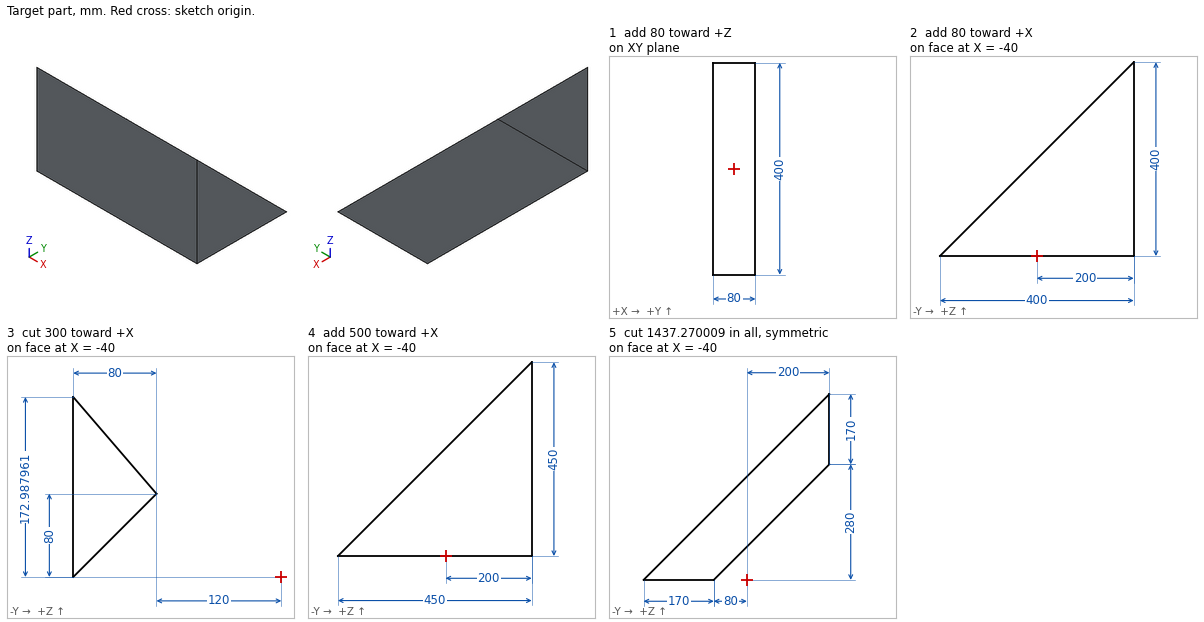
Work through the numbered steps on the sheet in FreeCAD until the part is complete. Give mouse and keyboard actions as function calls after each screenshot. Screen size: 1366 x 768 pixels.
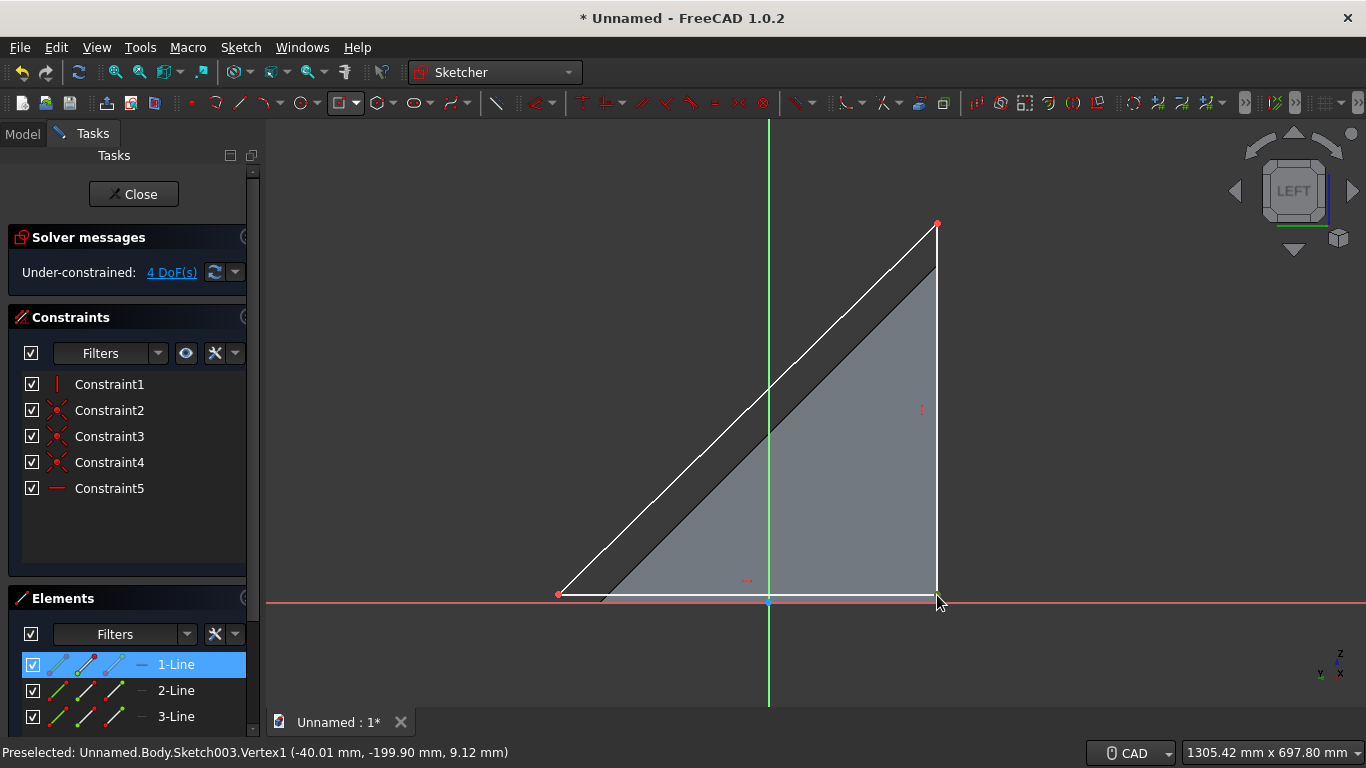
click(359, 603)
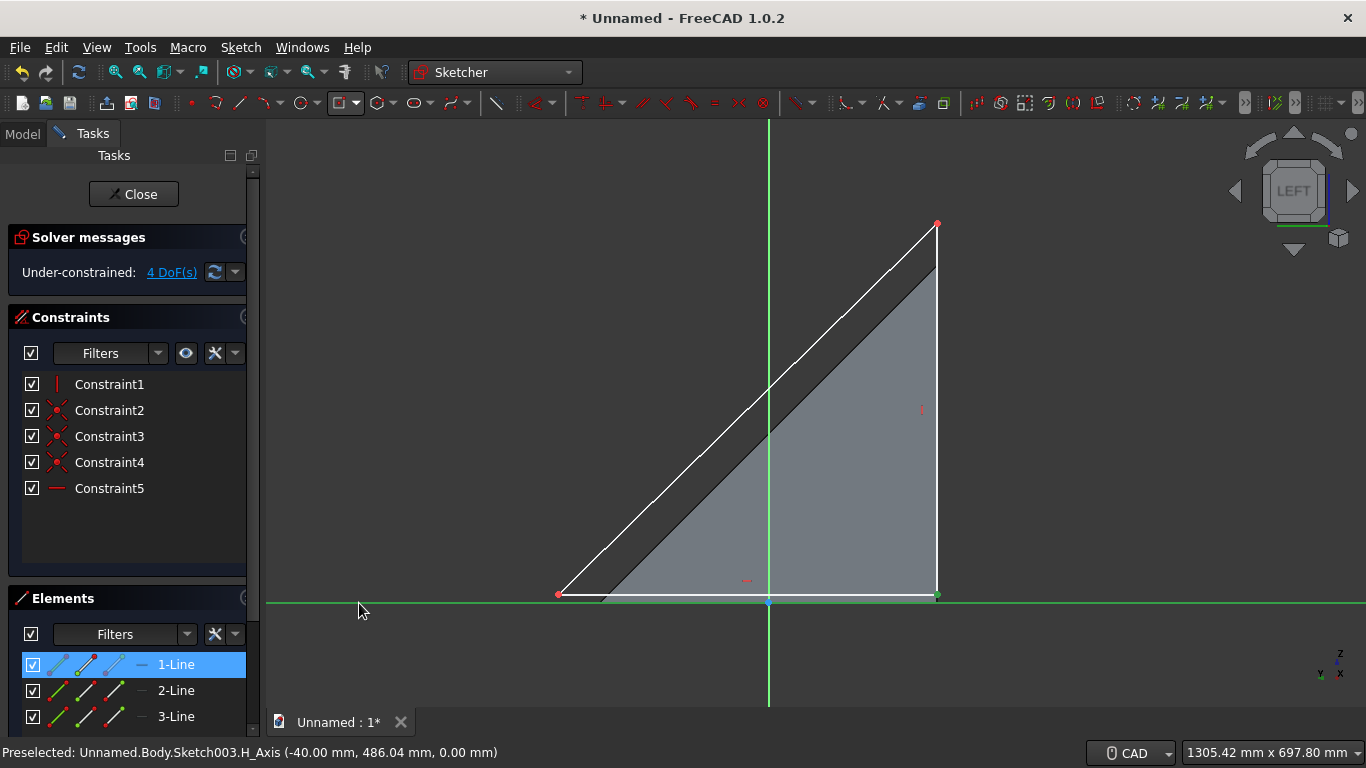
click(582, 104)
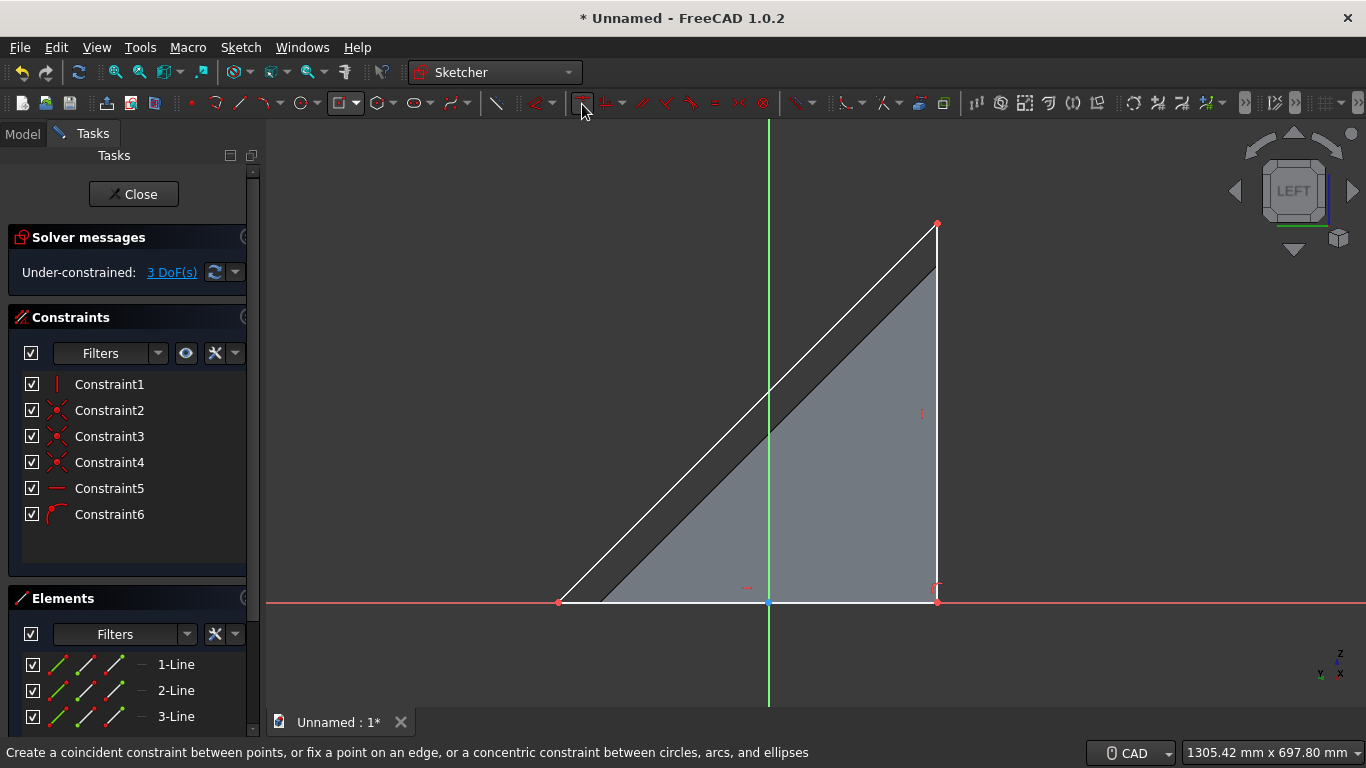
click(536, 104)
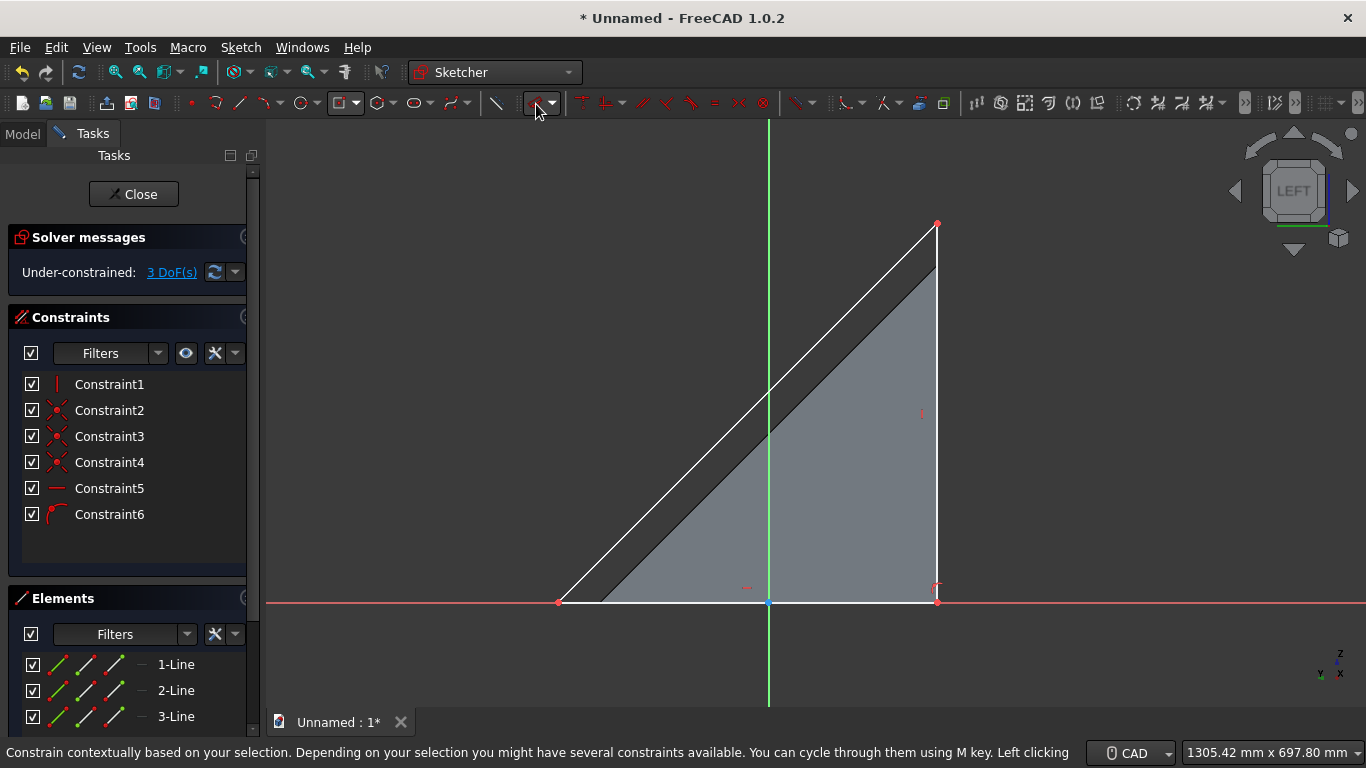
click(937, 489)
click(971, 413)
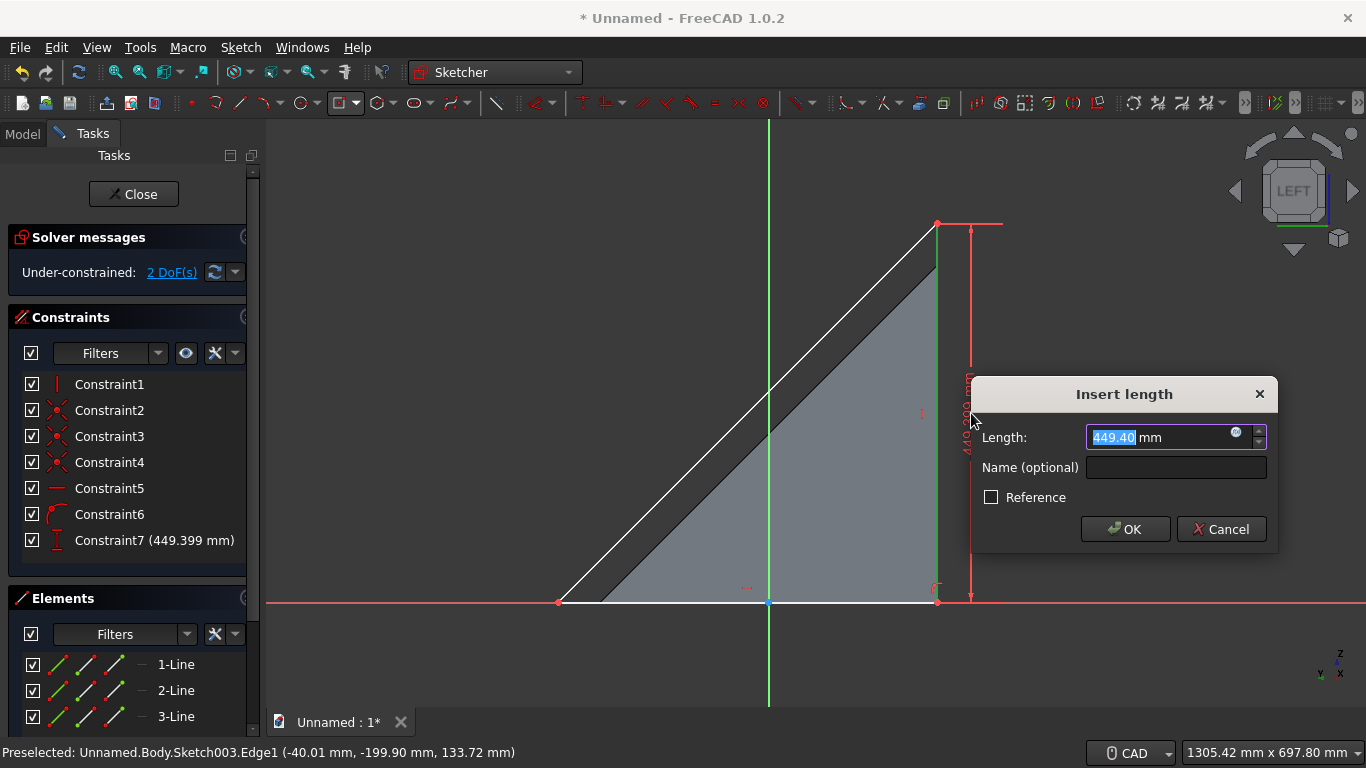
text(450)
key(Return)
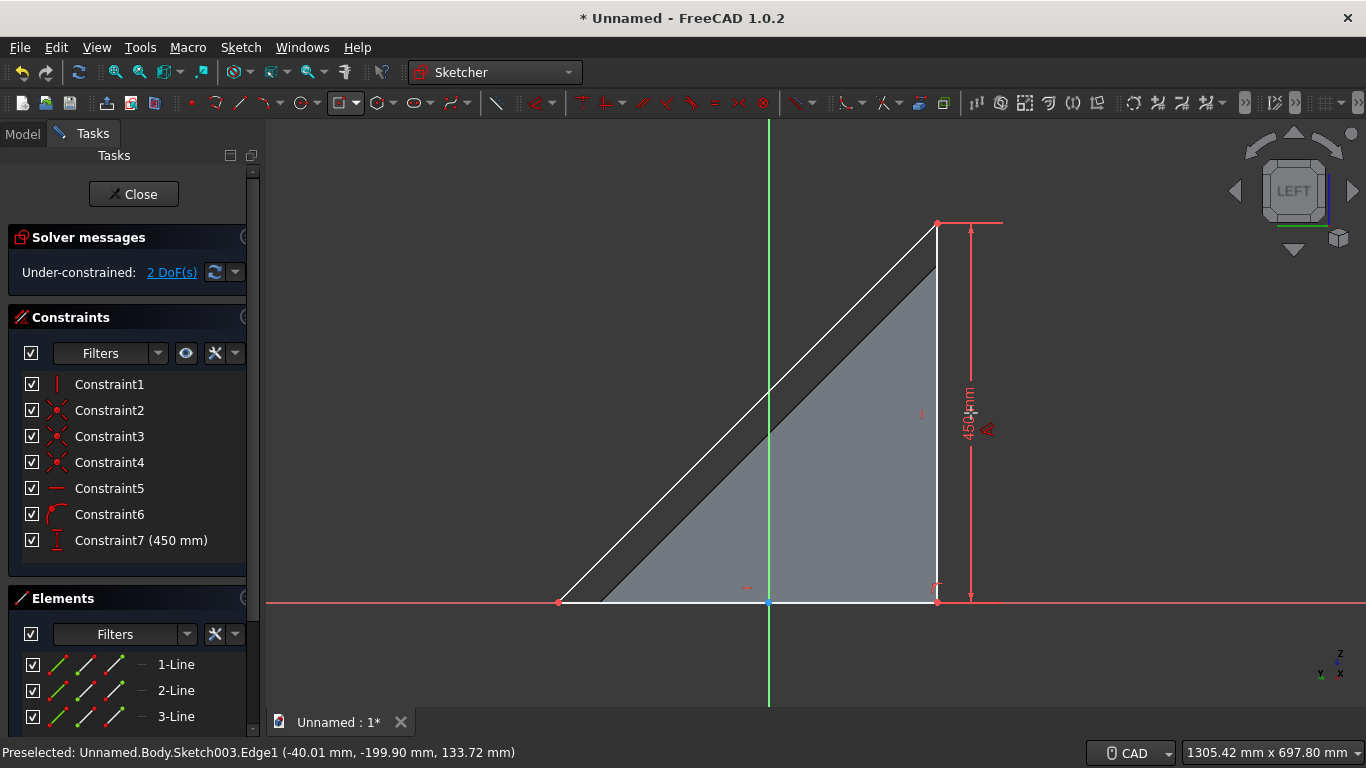
click(672, 603)
click(748, 637)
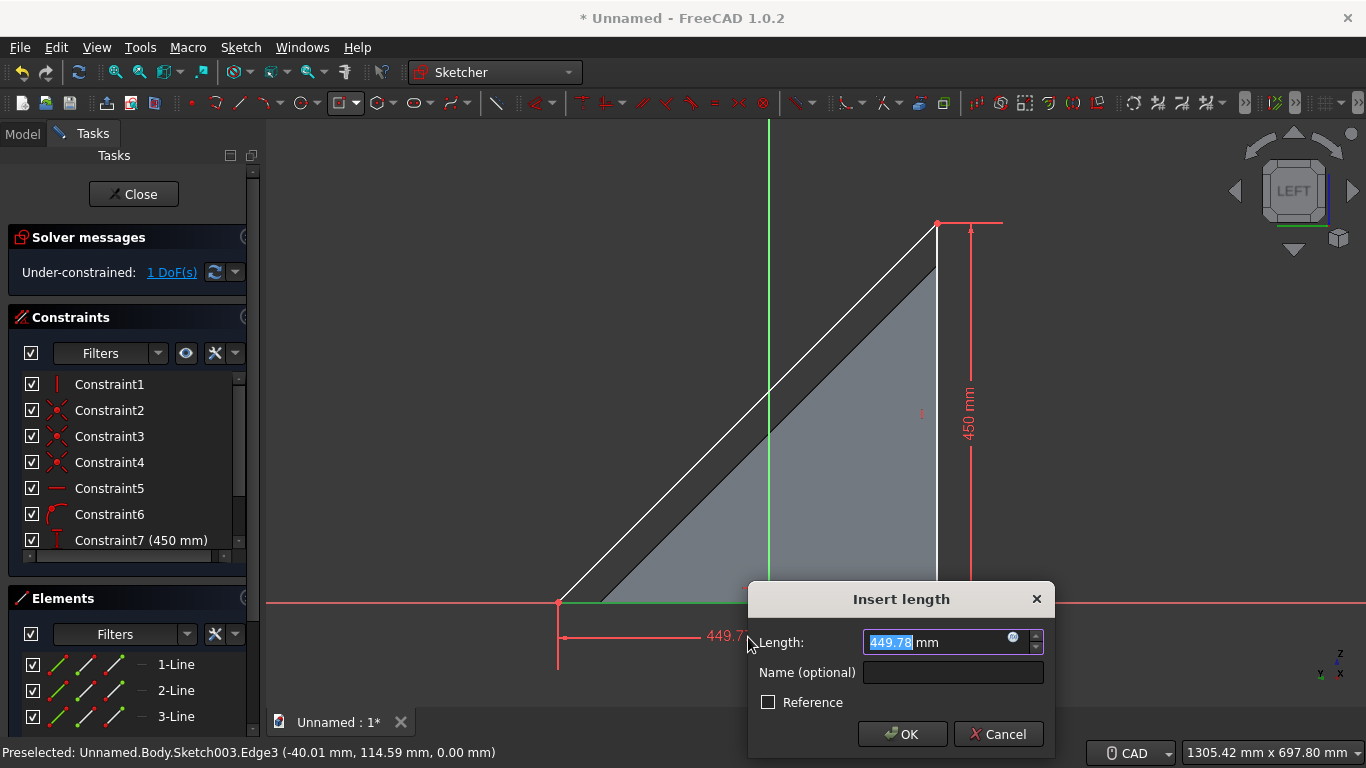
text(450)
key(Return)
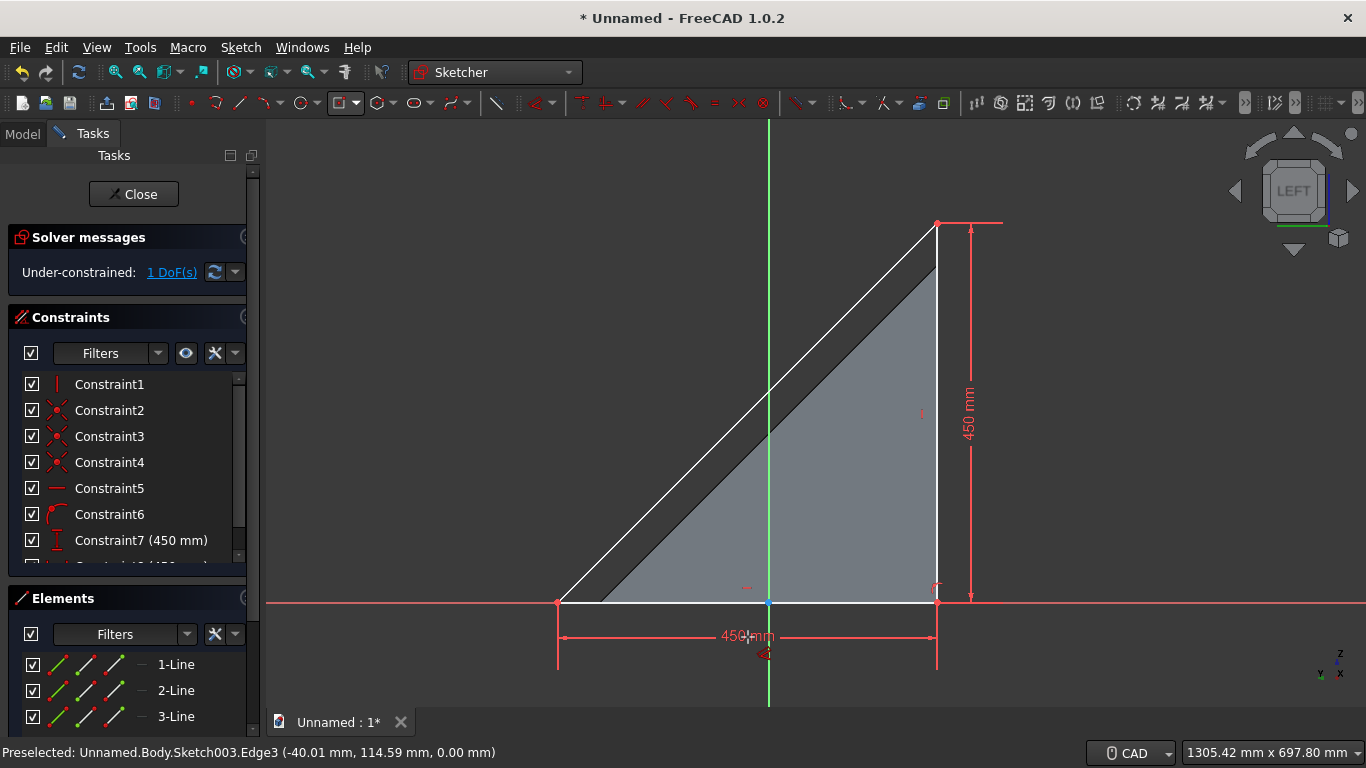
click(937, 603)
click(853, 637)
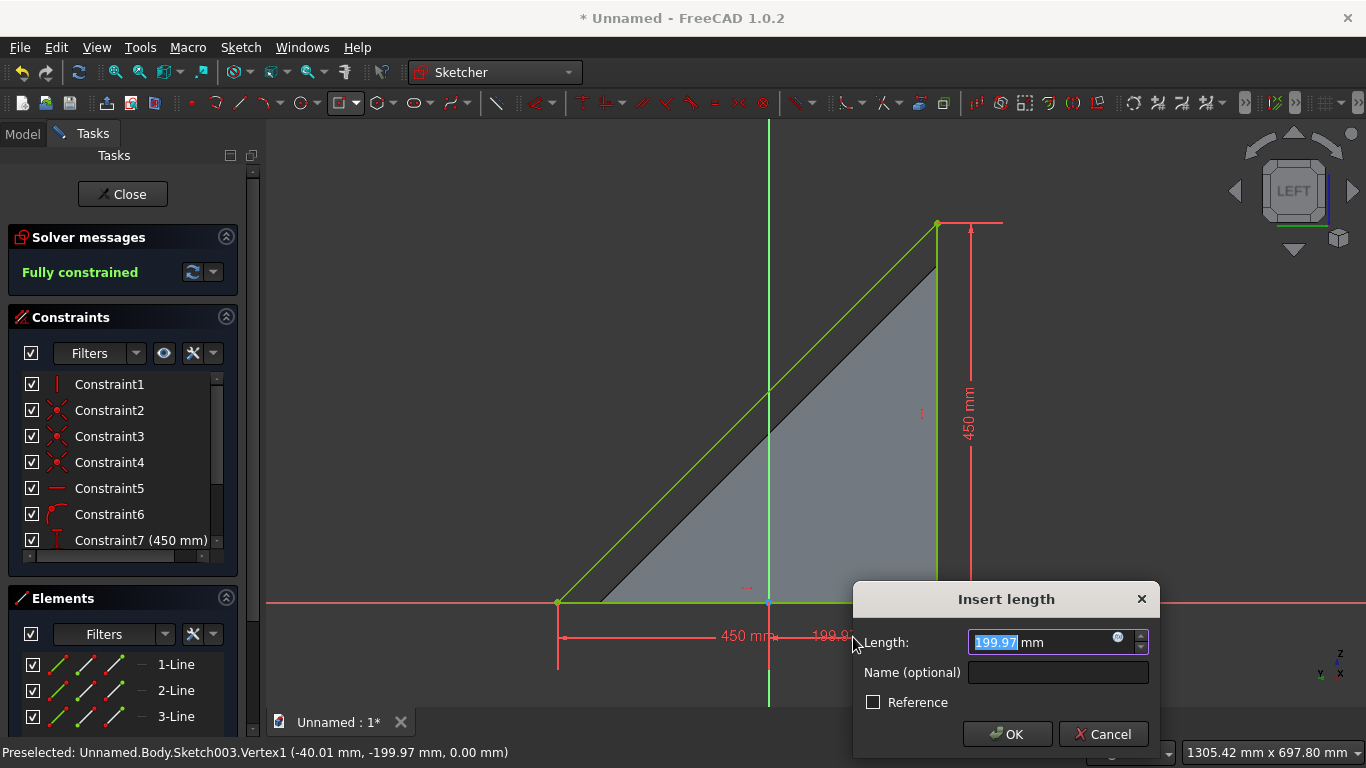
text(200)
key(Return)
key(Escape)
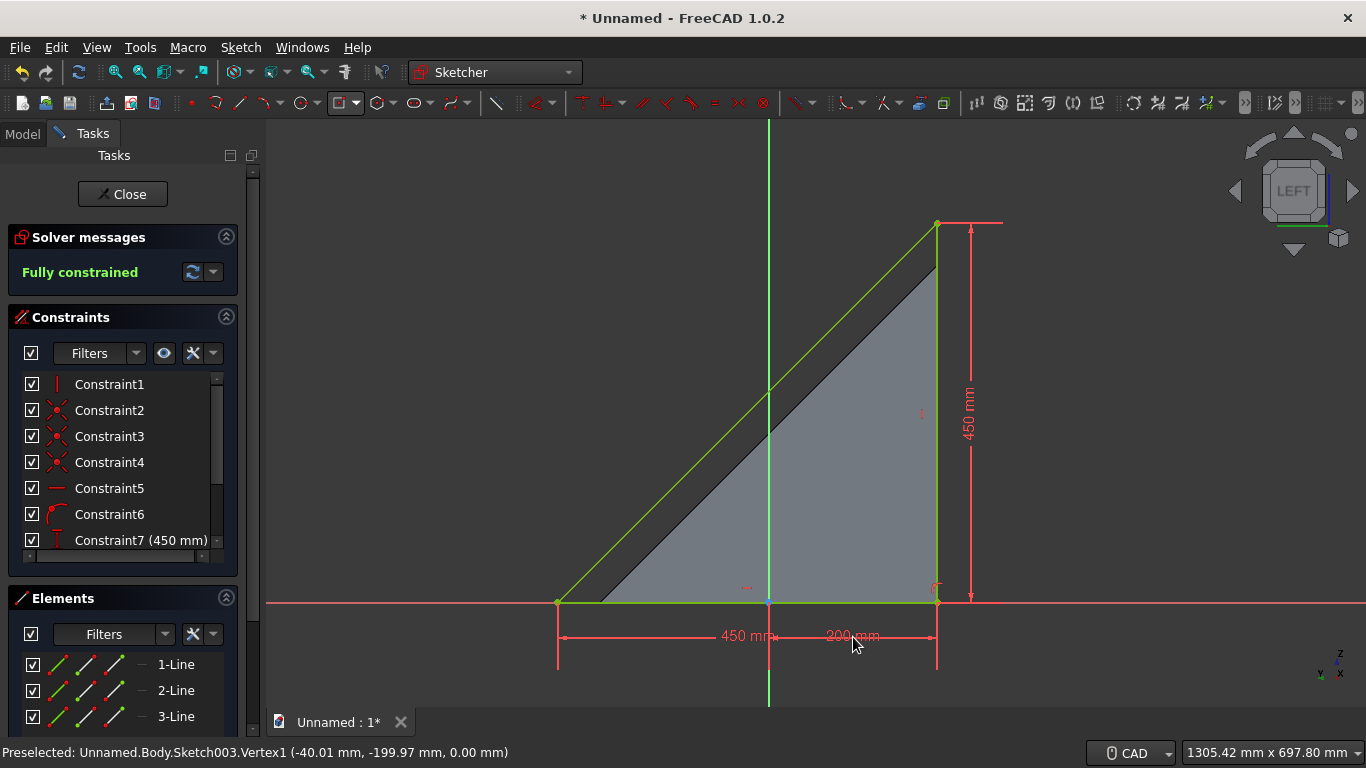
click(123, 194)